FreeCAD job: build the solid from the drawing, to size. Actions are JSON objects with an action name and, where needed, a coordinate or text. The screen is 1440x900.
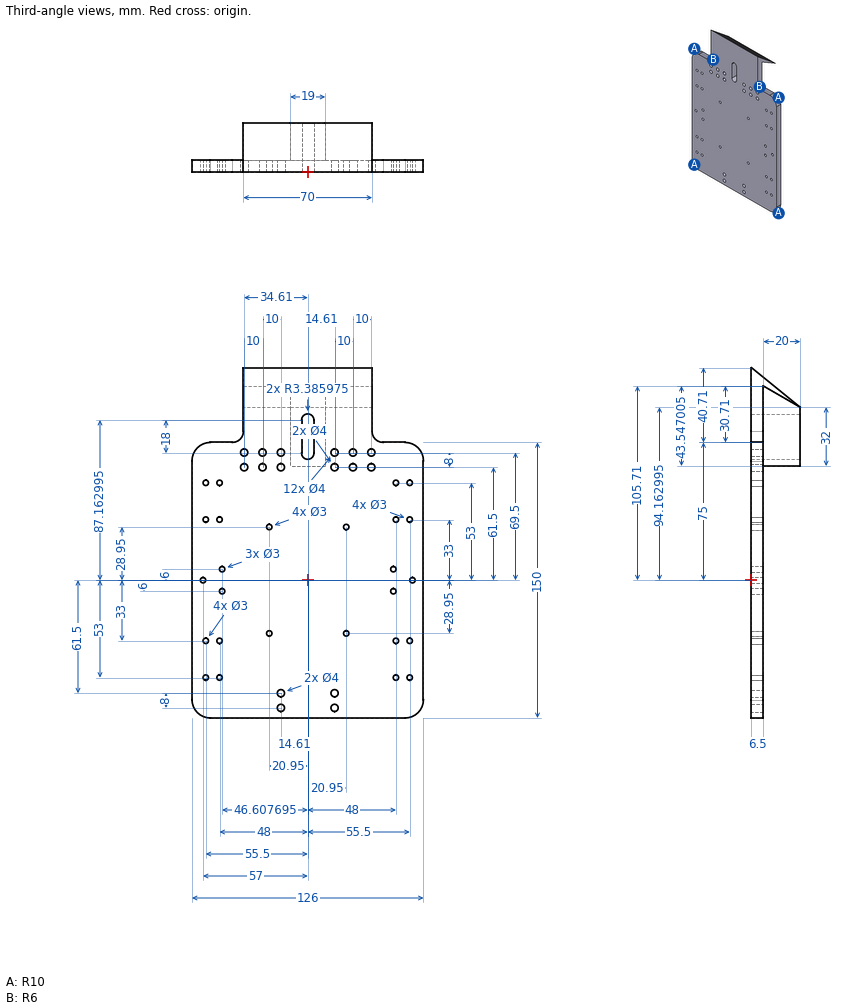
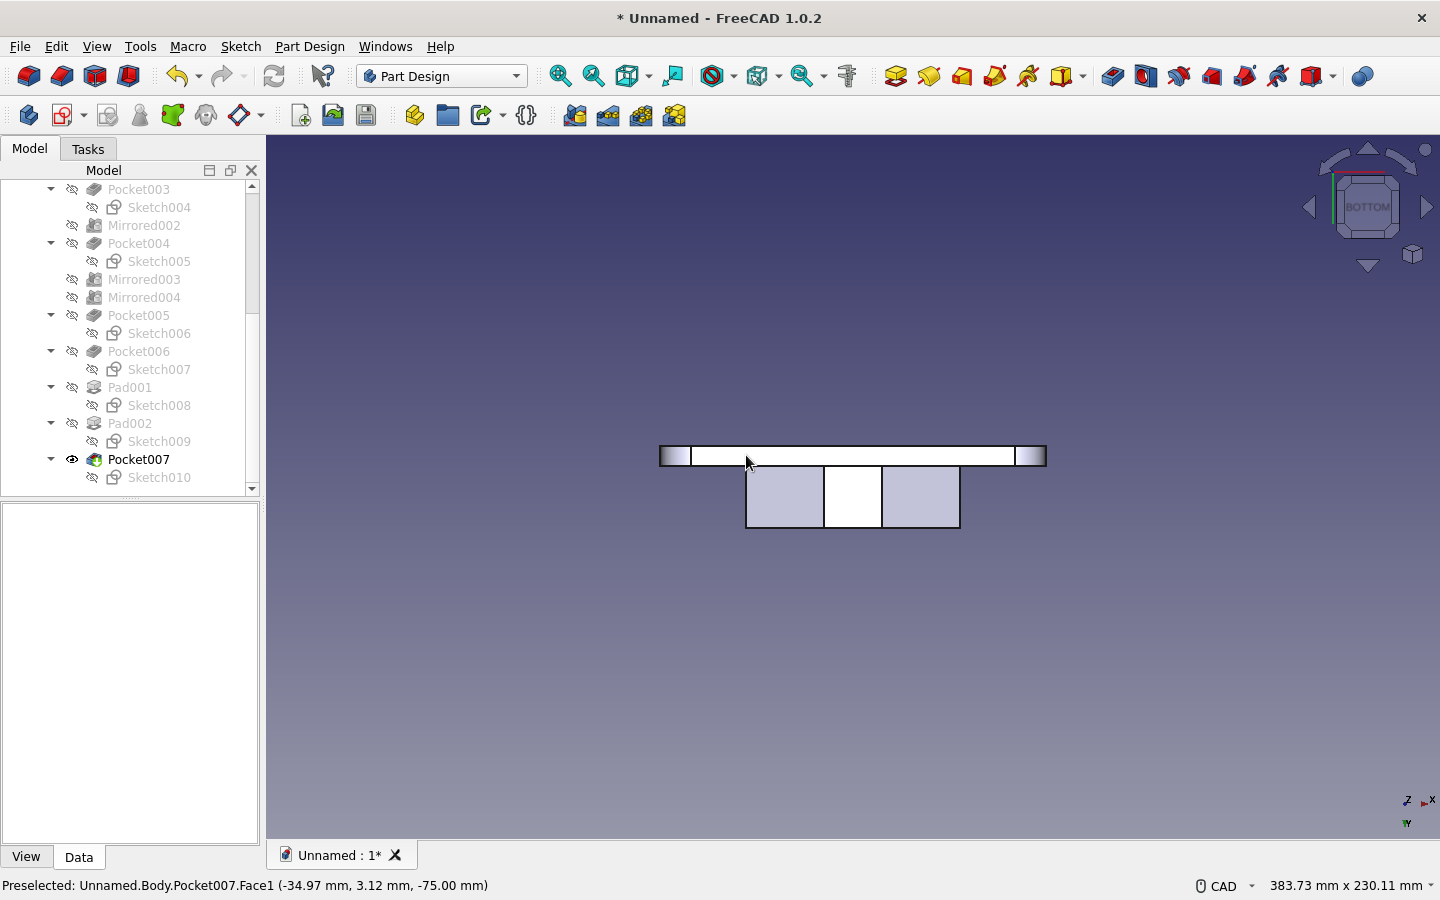
{"action": "key", "text": "4"}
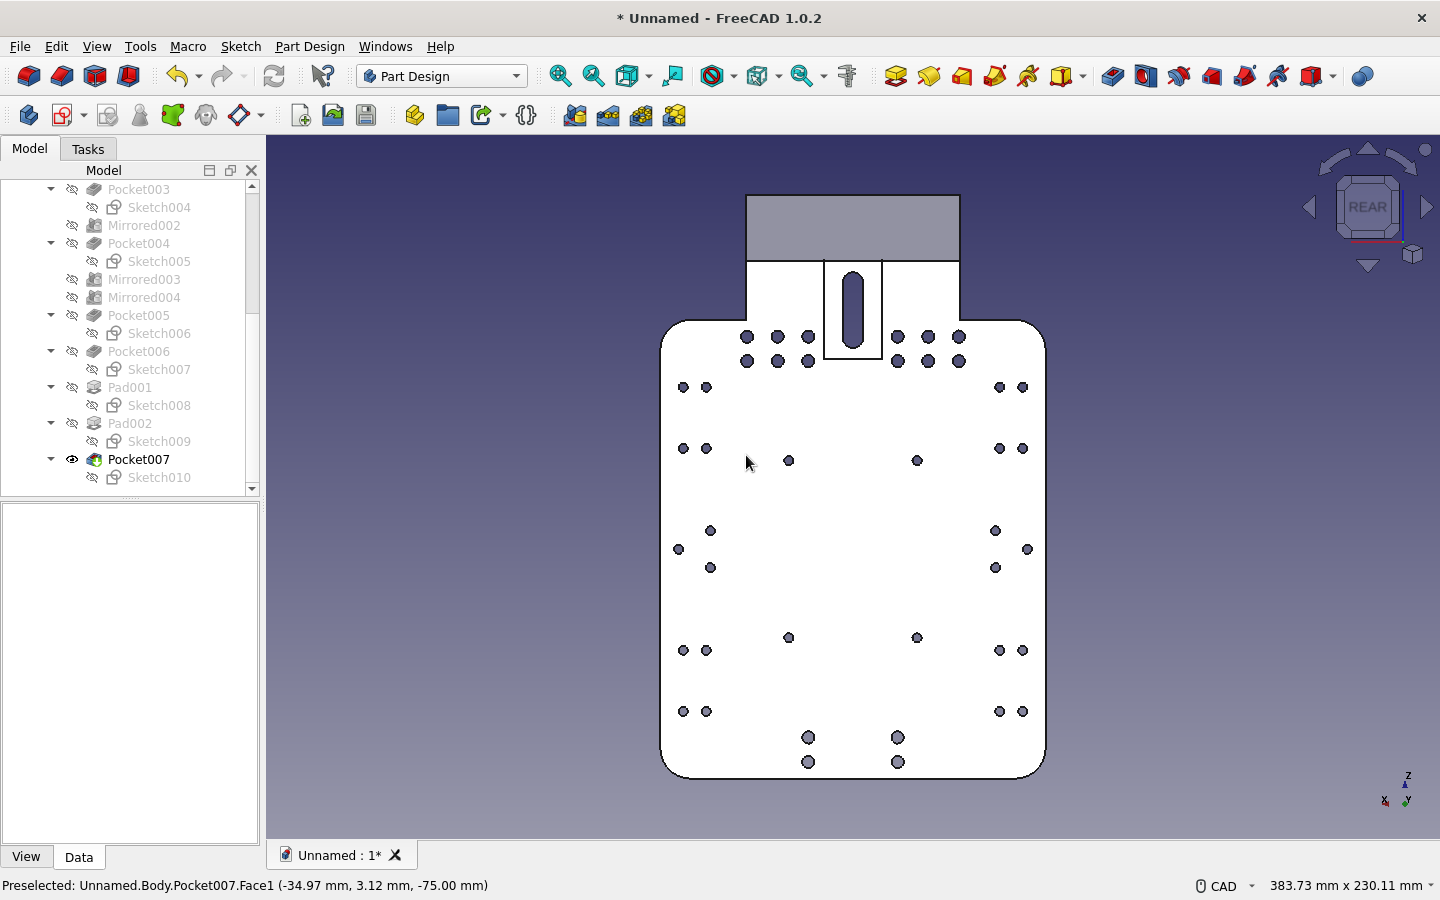
{"action": "scroll", "coordinate": [960, 319], "scroll_direction": "up", "scroll_amount": 4}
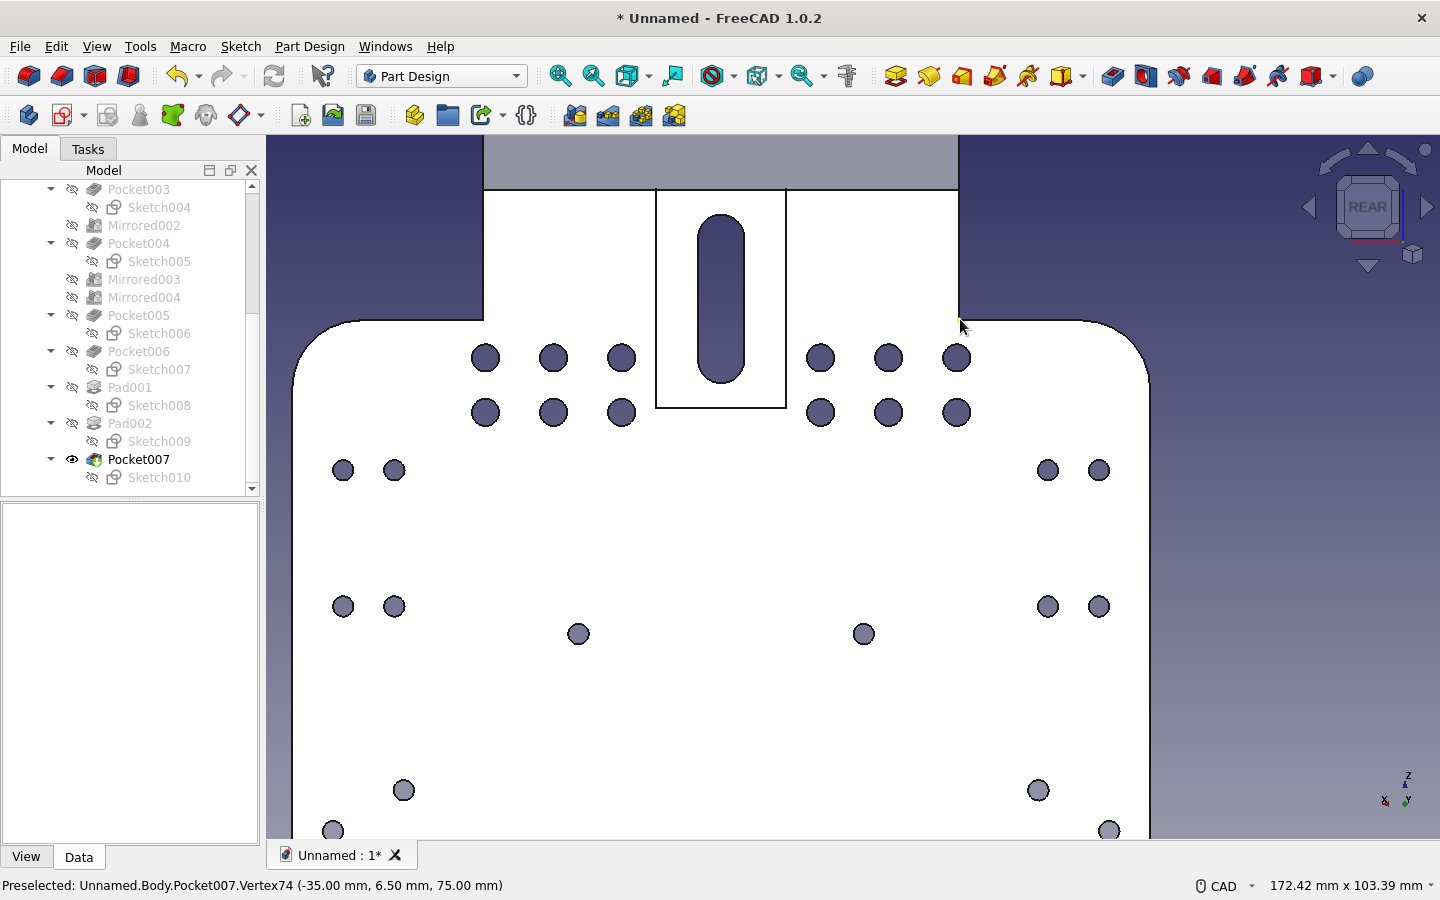
{"action": "left_click", "coordinate": [561, 76]}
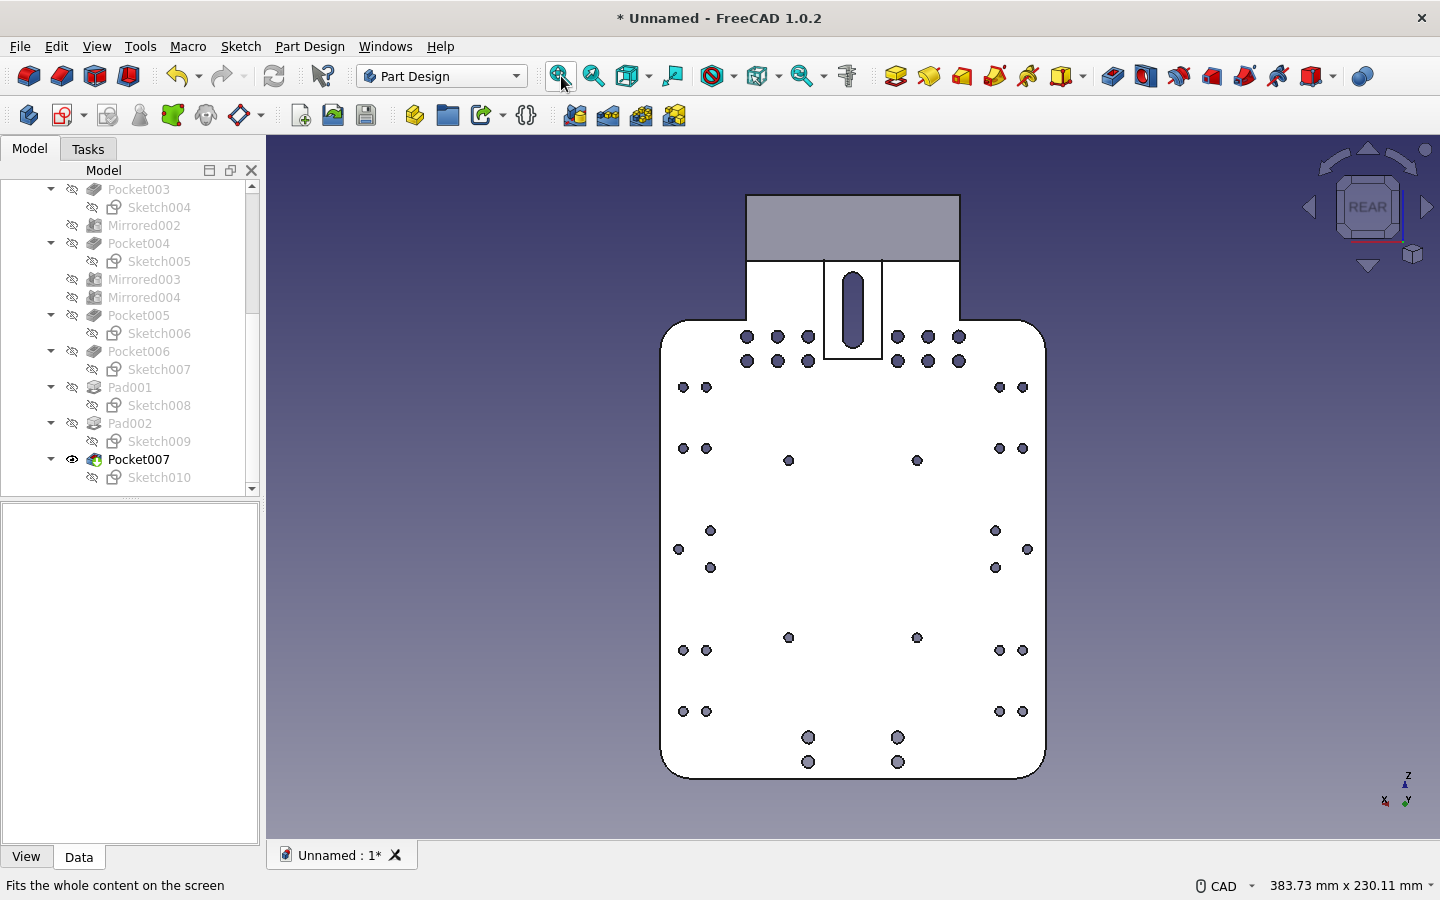
{"action": "key", "text": "6"}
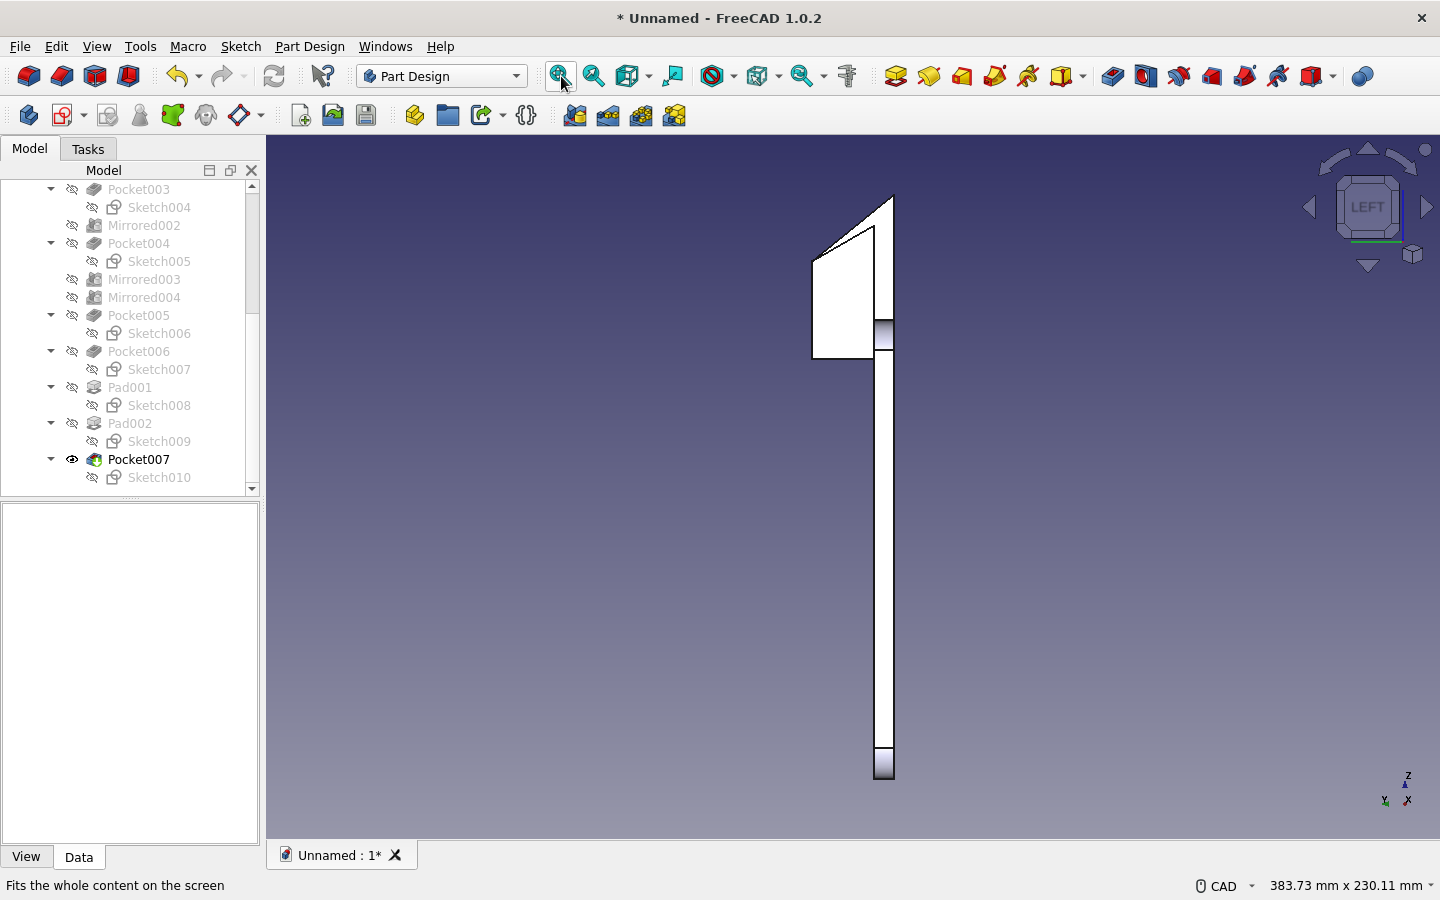
{"action": "scroll", "coordinate": [884, 319], "scroll_direction": "up", "scroll_amount": 4}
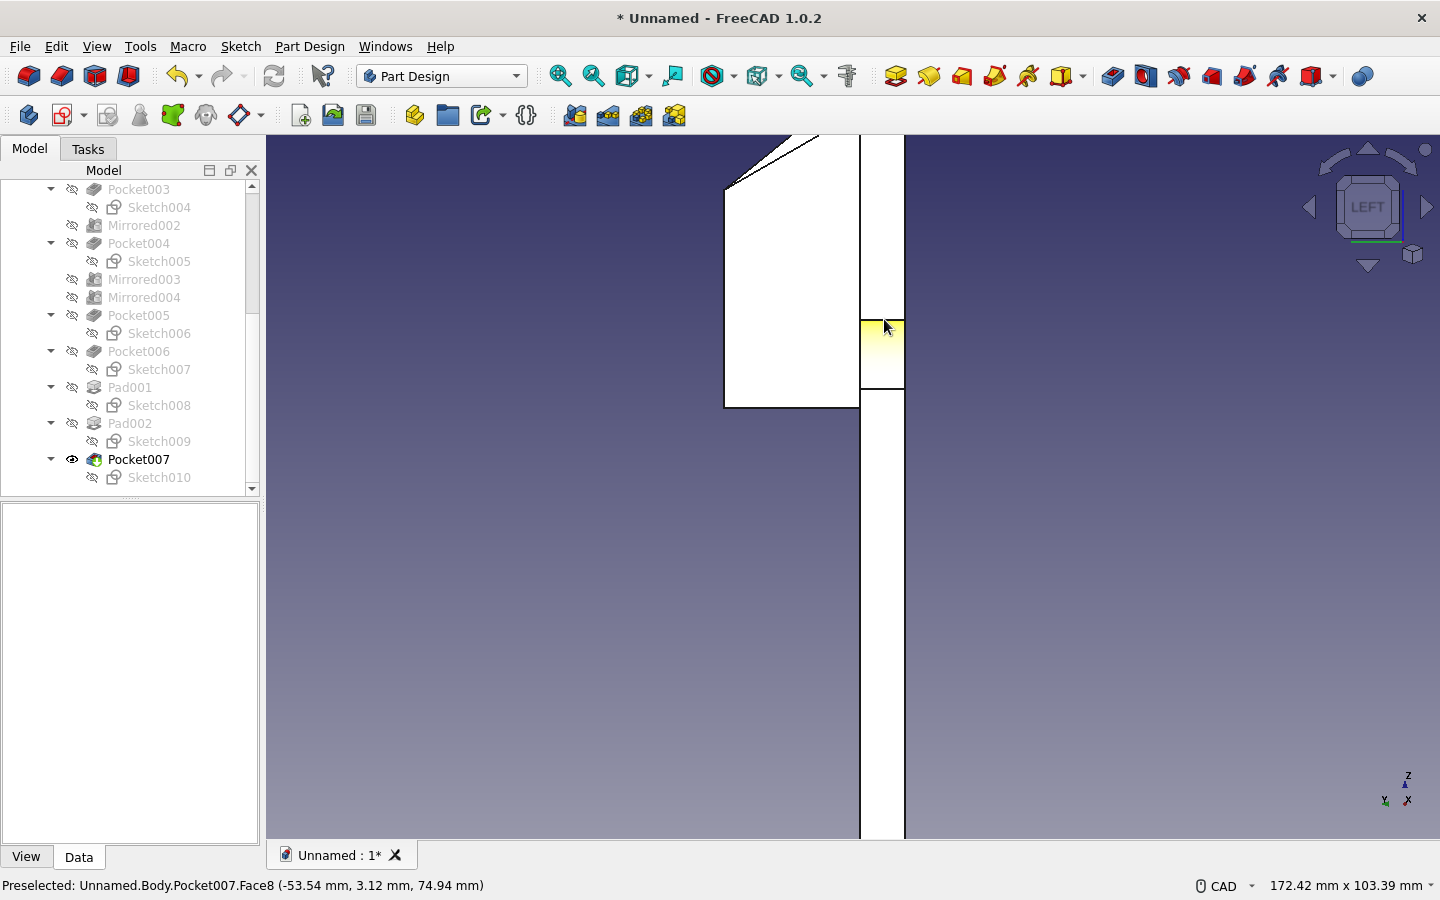
{"action": "left_click", "coordinate": [561, 76]}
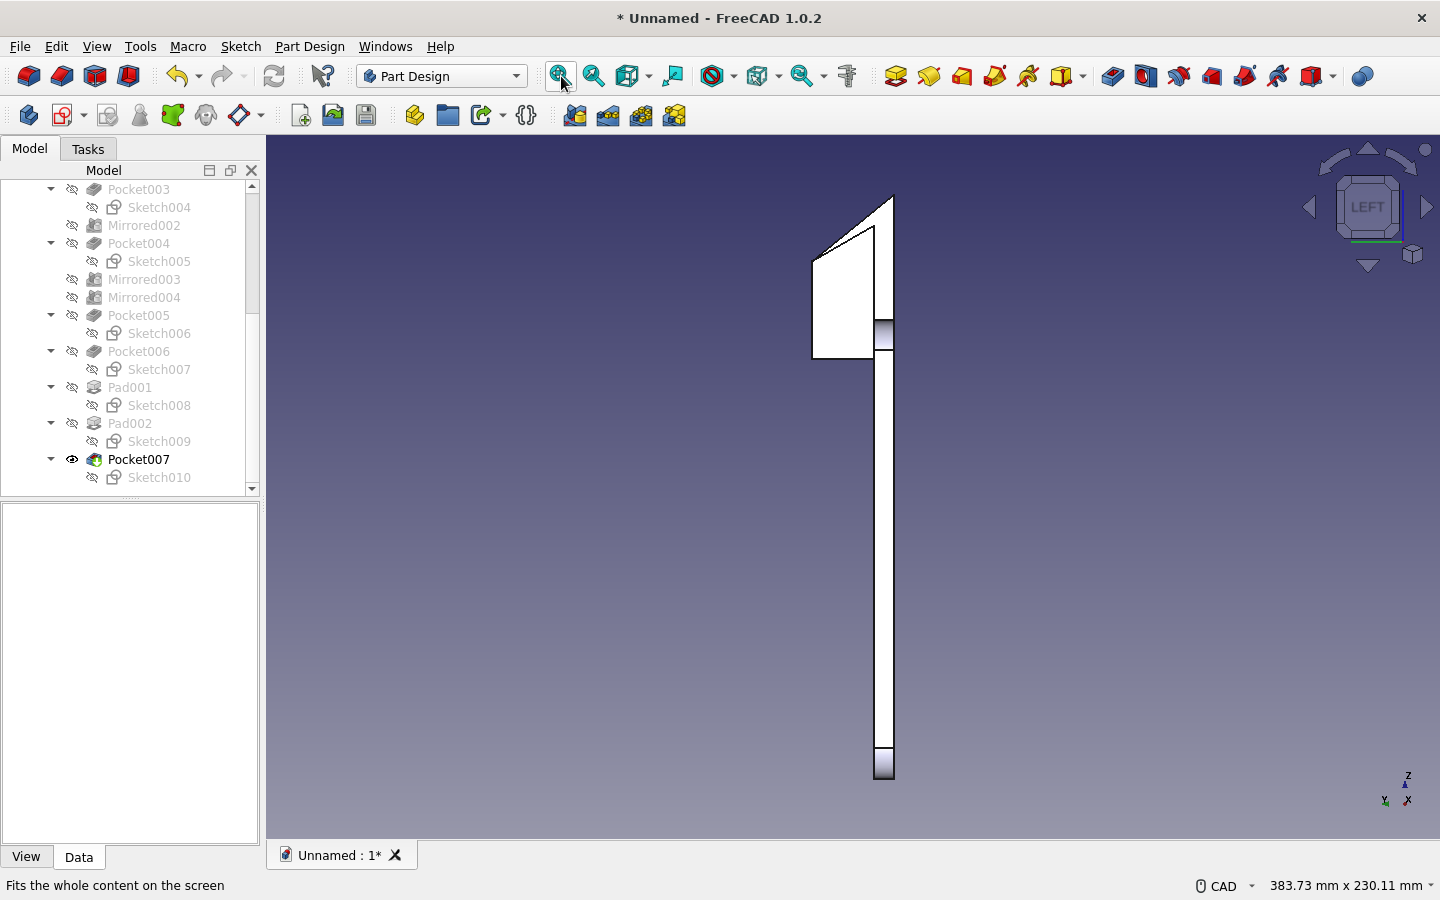
{"action": "key", "text": "v 3"}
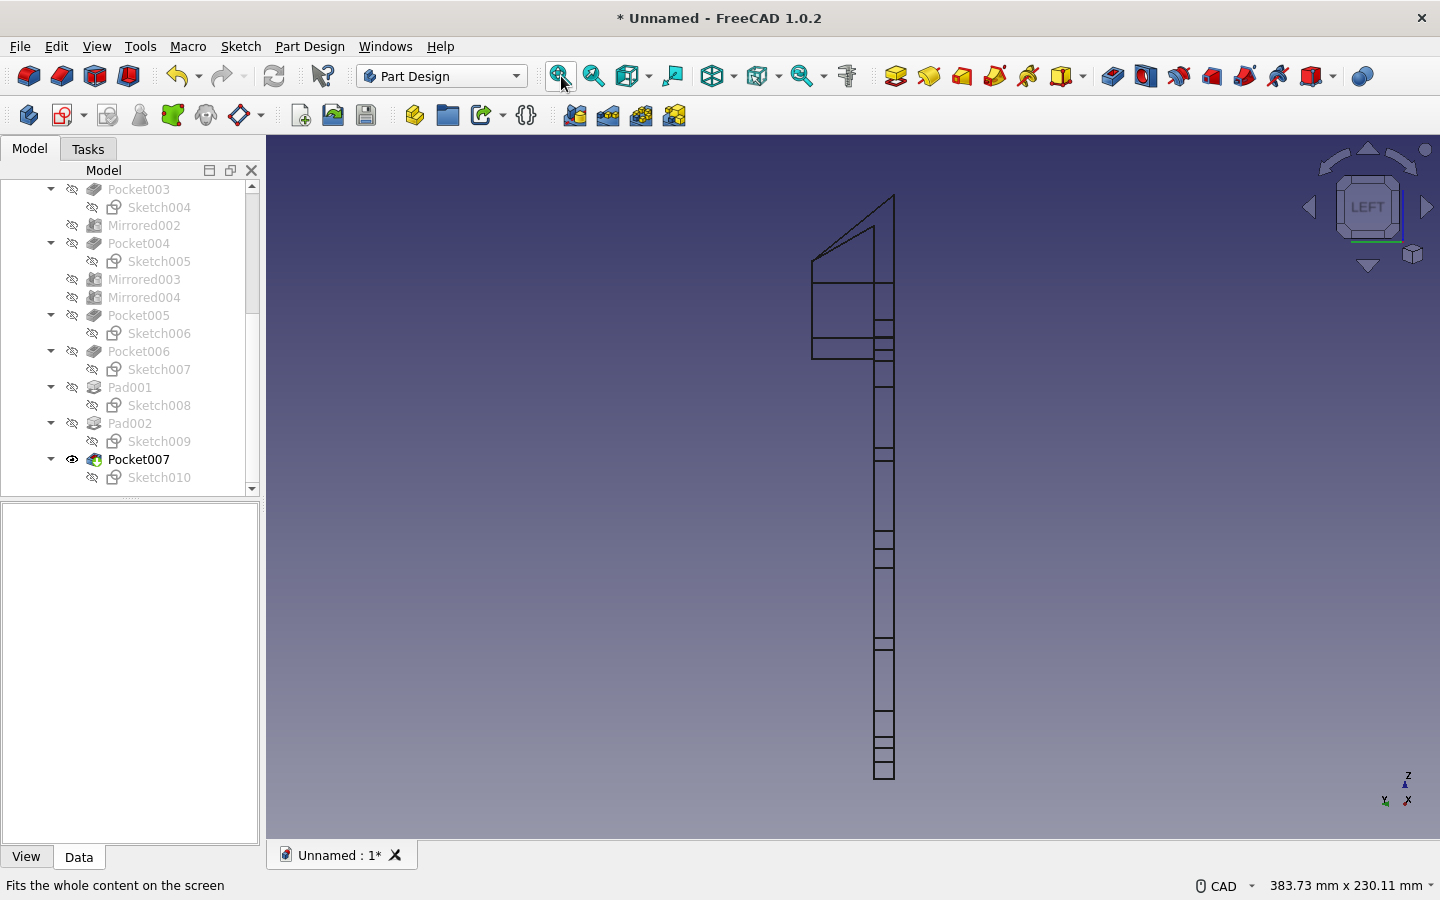
{"action": "key", "text": "0"}